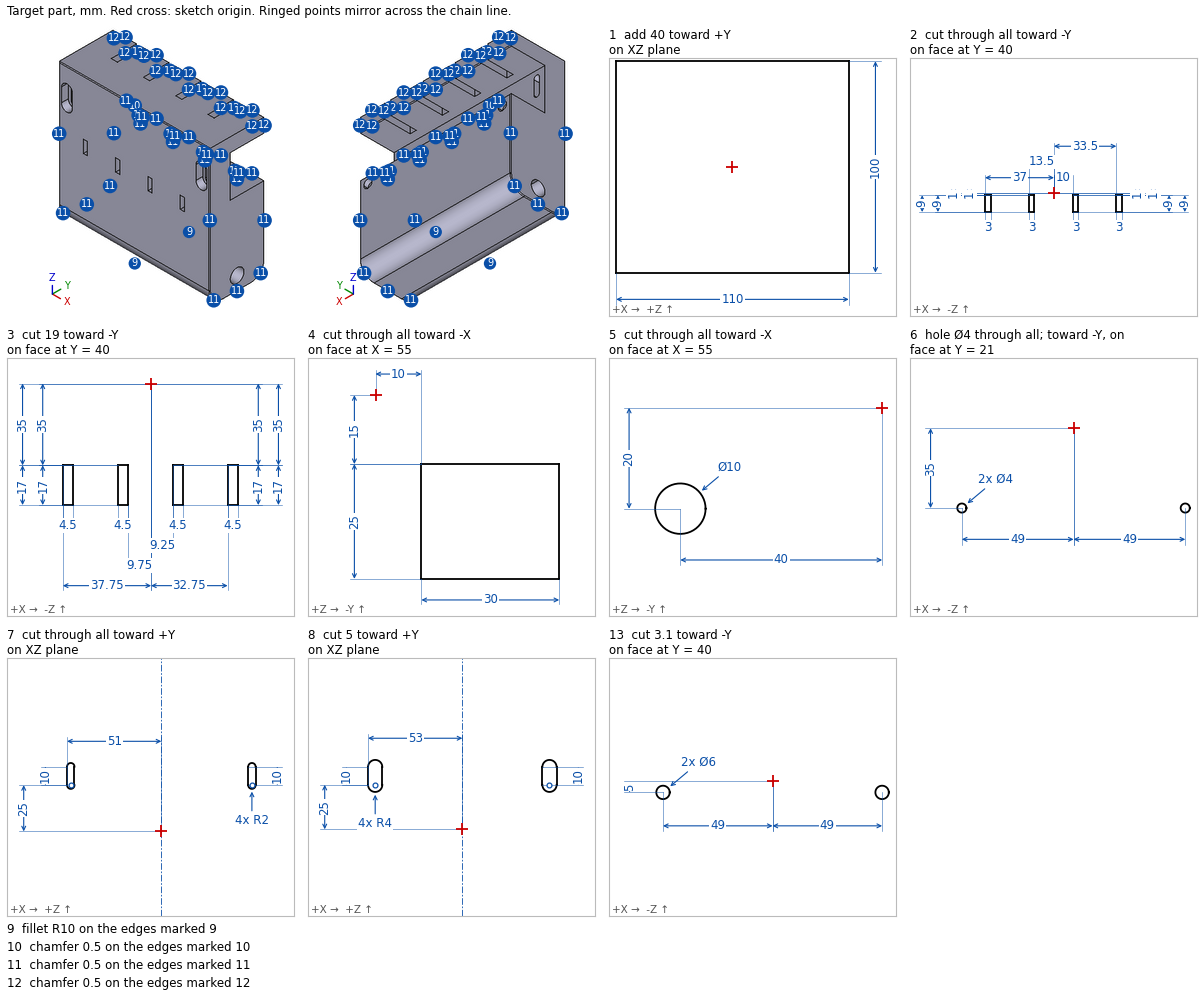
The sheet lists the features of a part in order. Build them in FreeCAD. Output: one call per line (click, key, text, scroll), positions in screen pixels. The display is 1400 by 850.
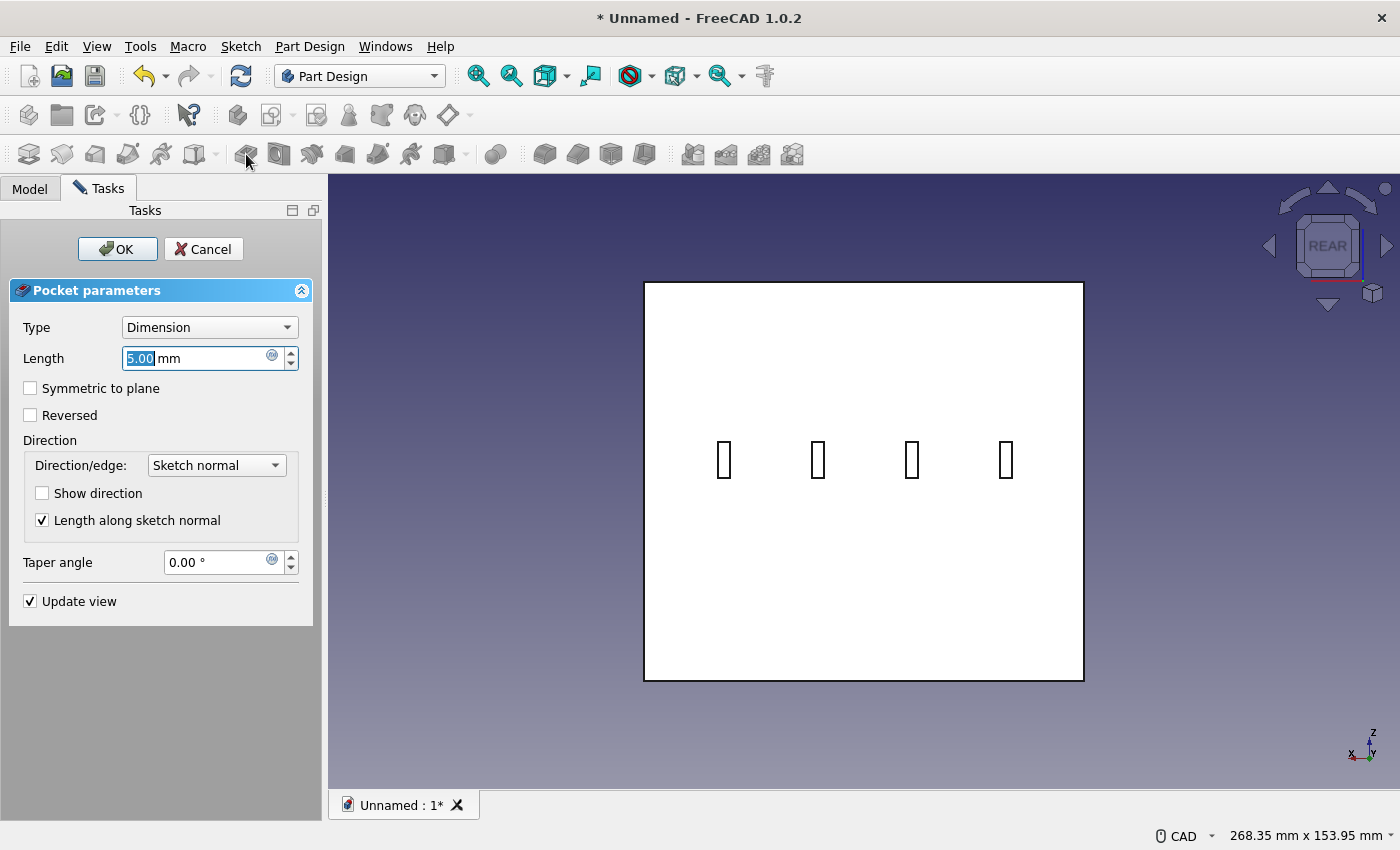
click(210, 328)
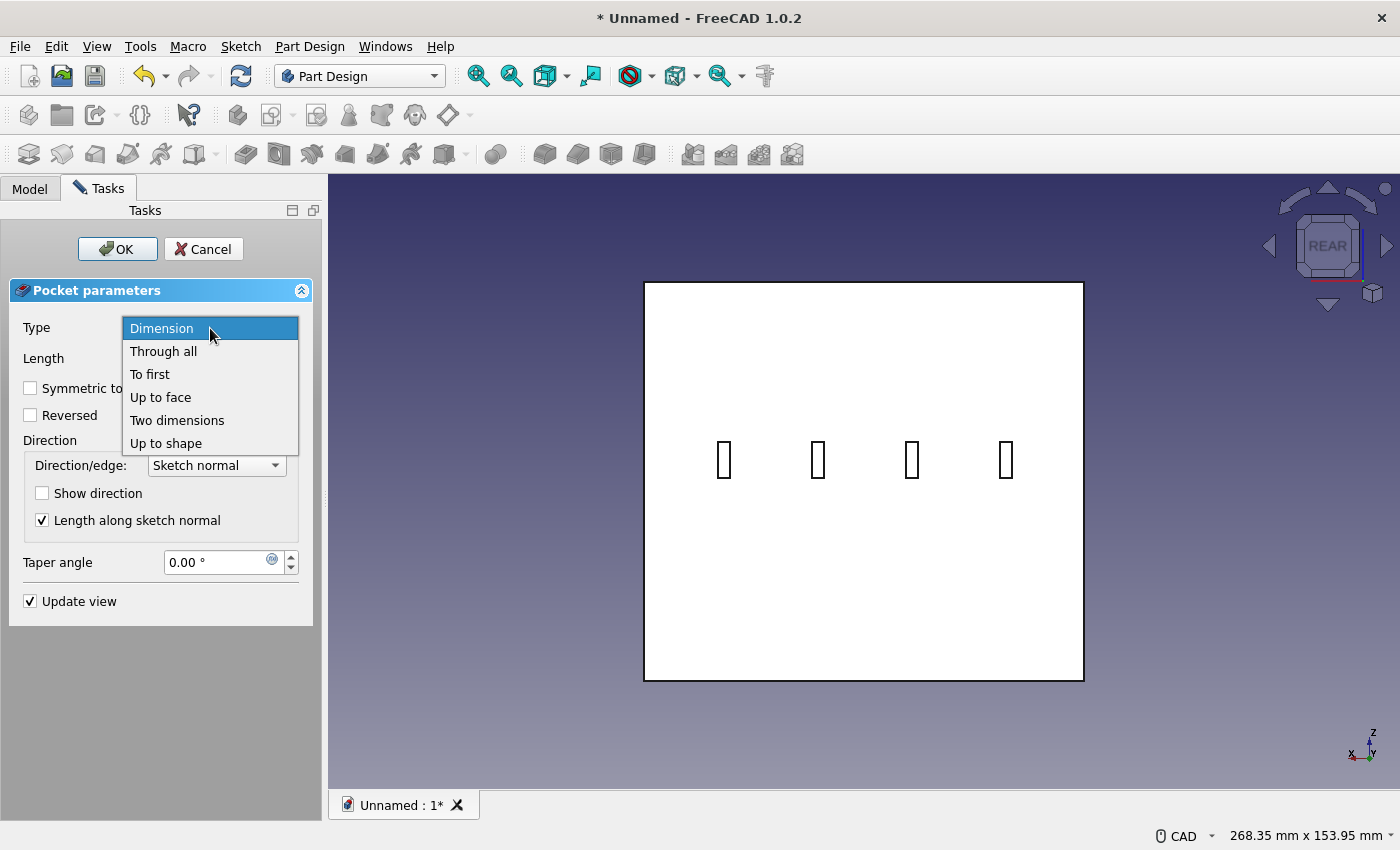
click(208, 352)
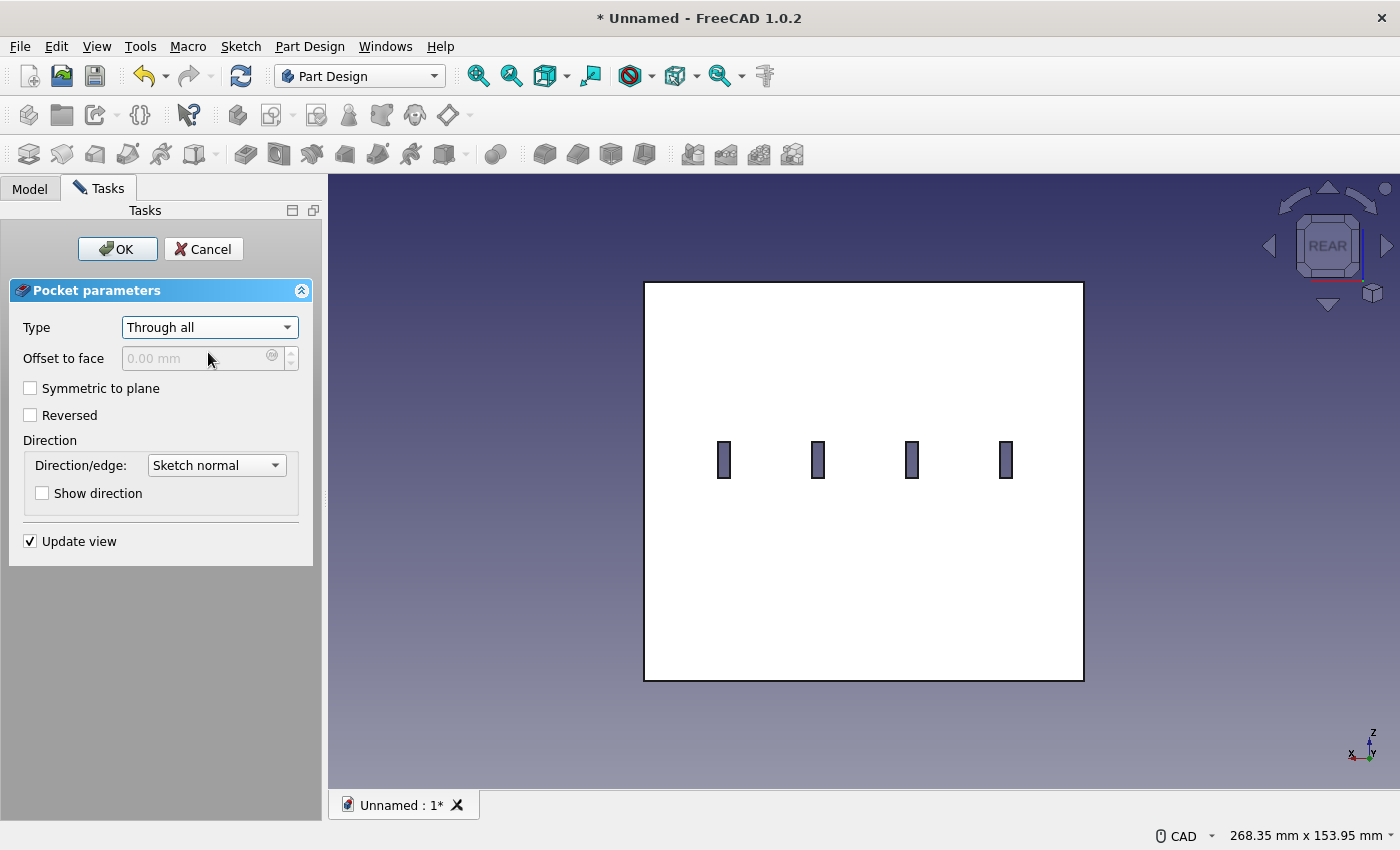
click(118, 249)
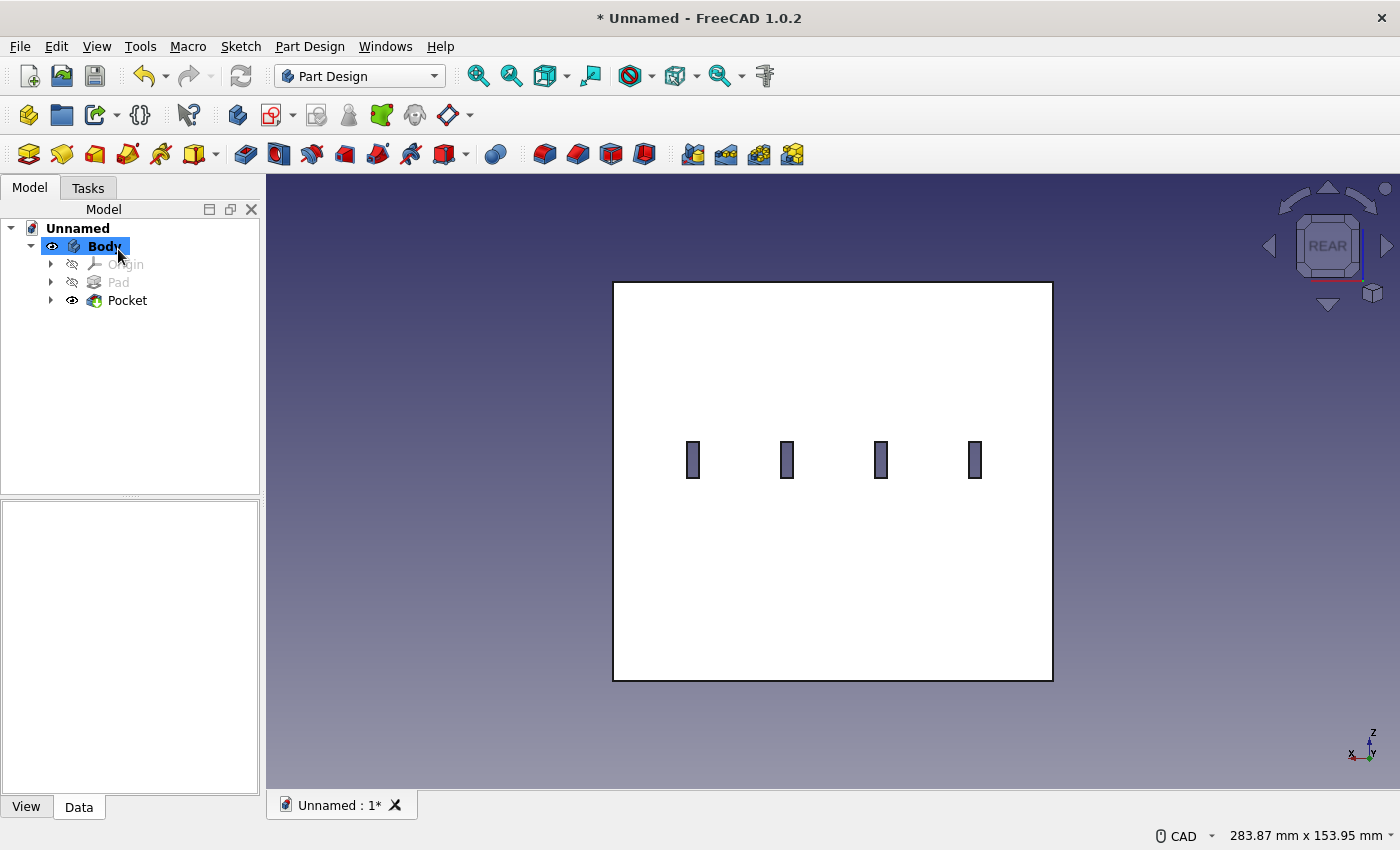
click(707, 595)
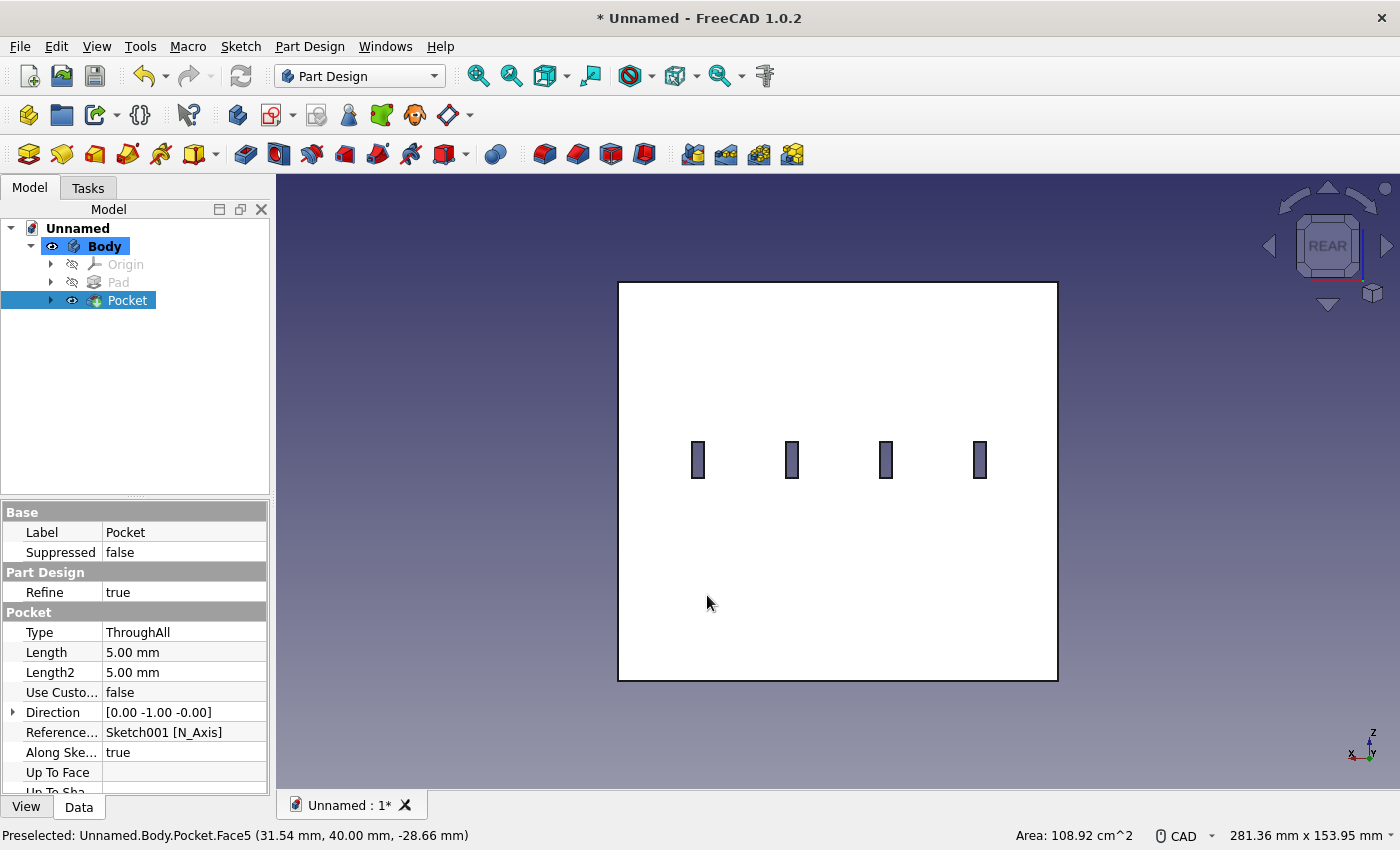
click(270, 116)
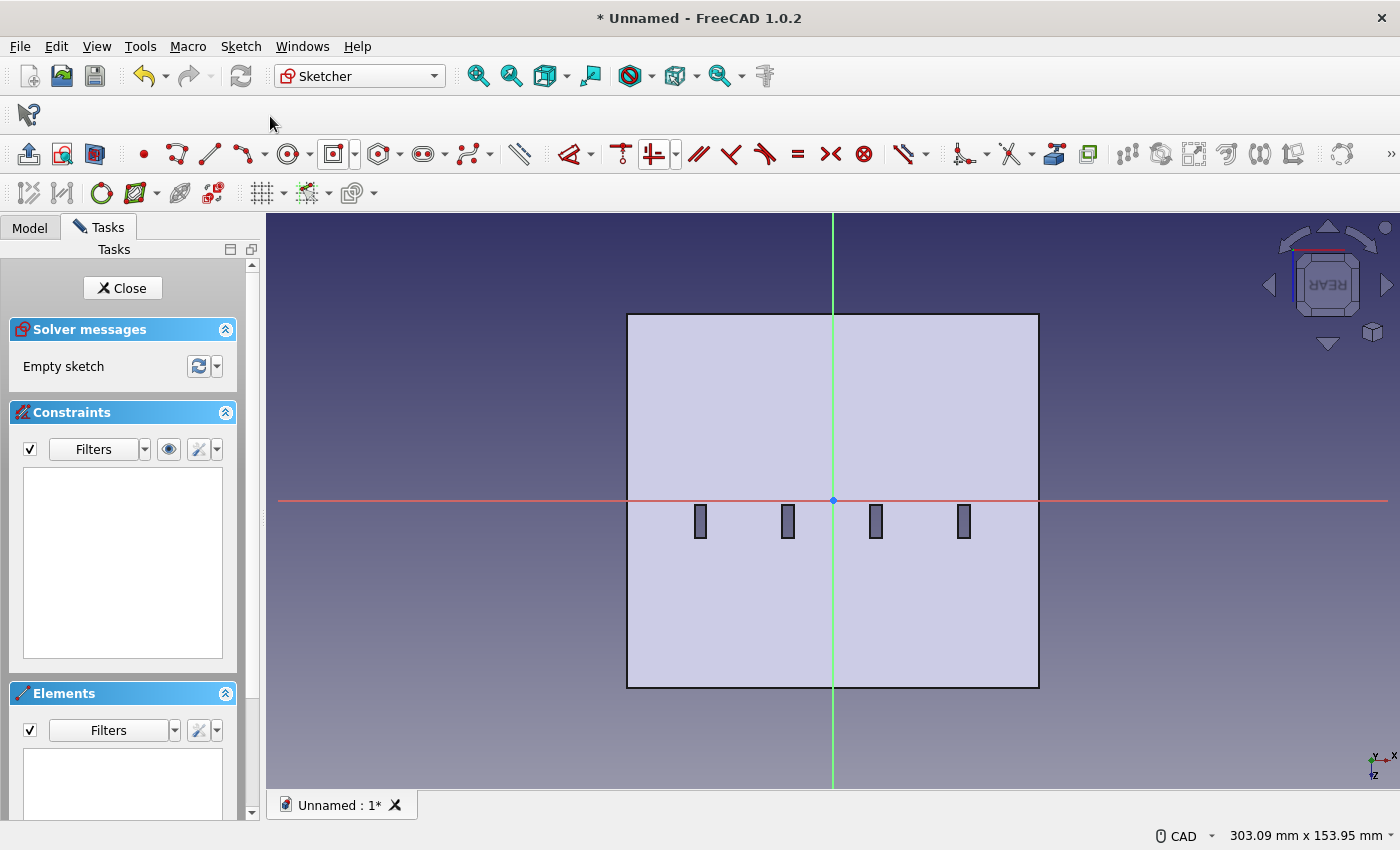
scroll(914, 717, up, 3)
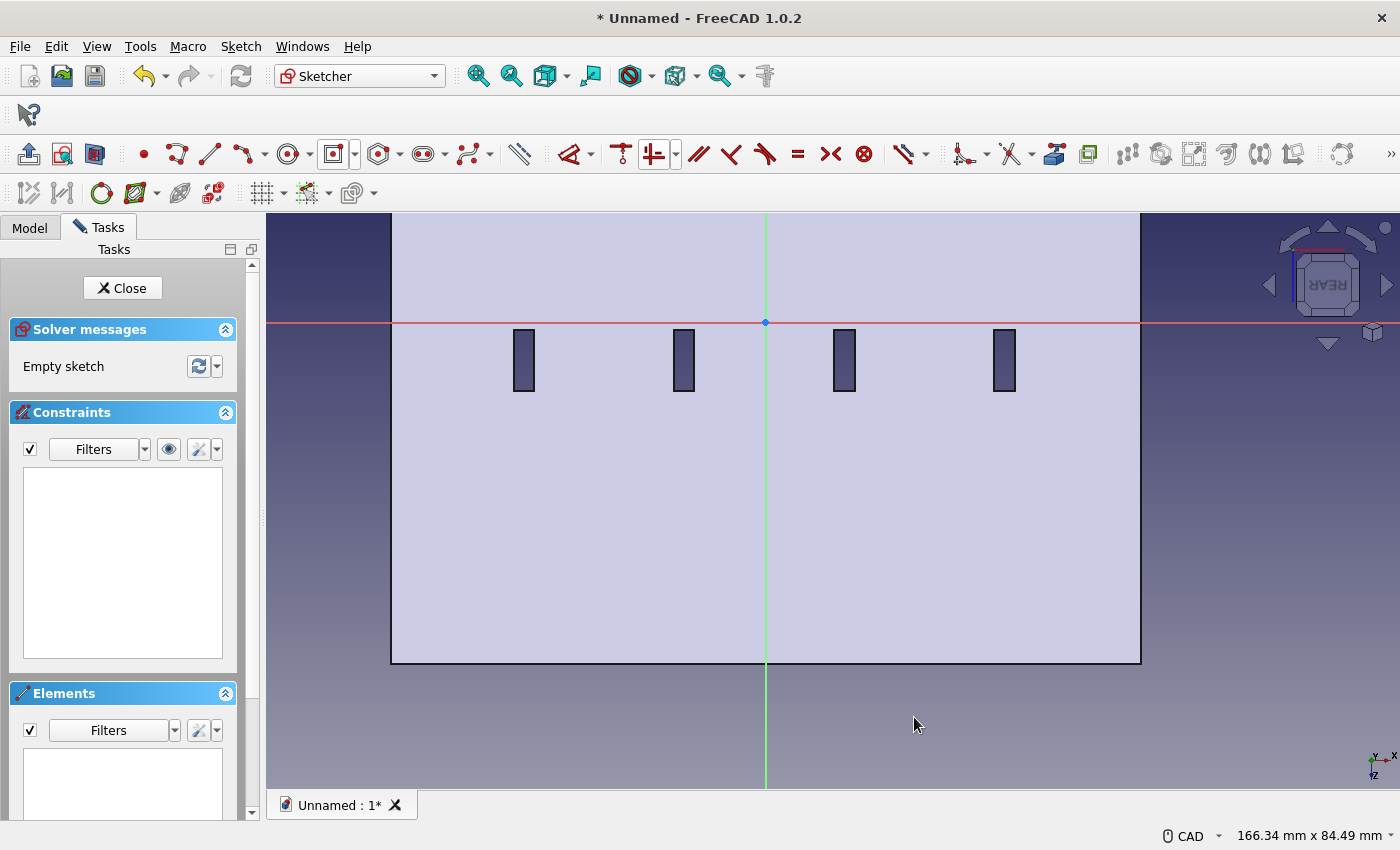
key(g)
key(r)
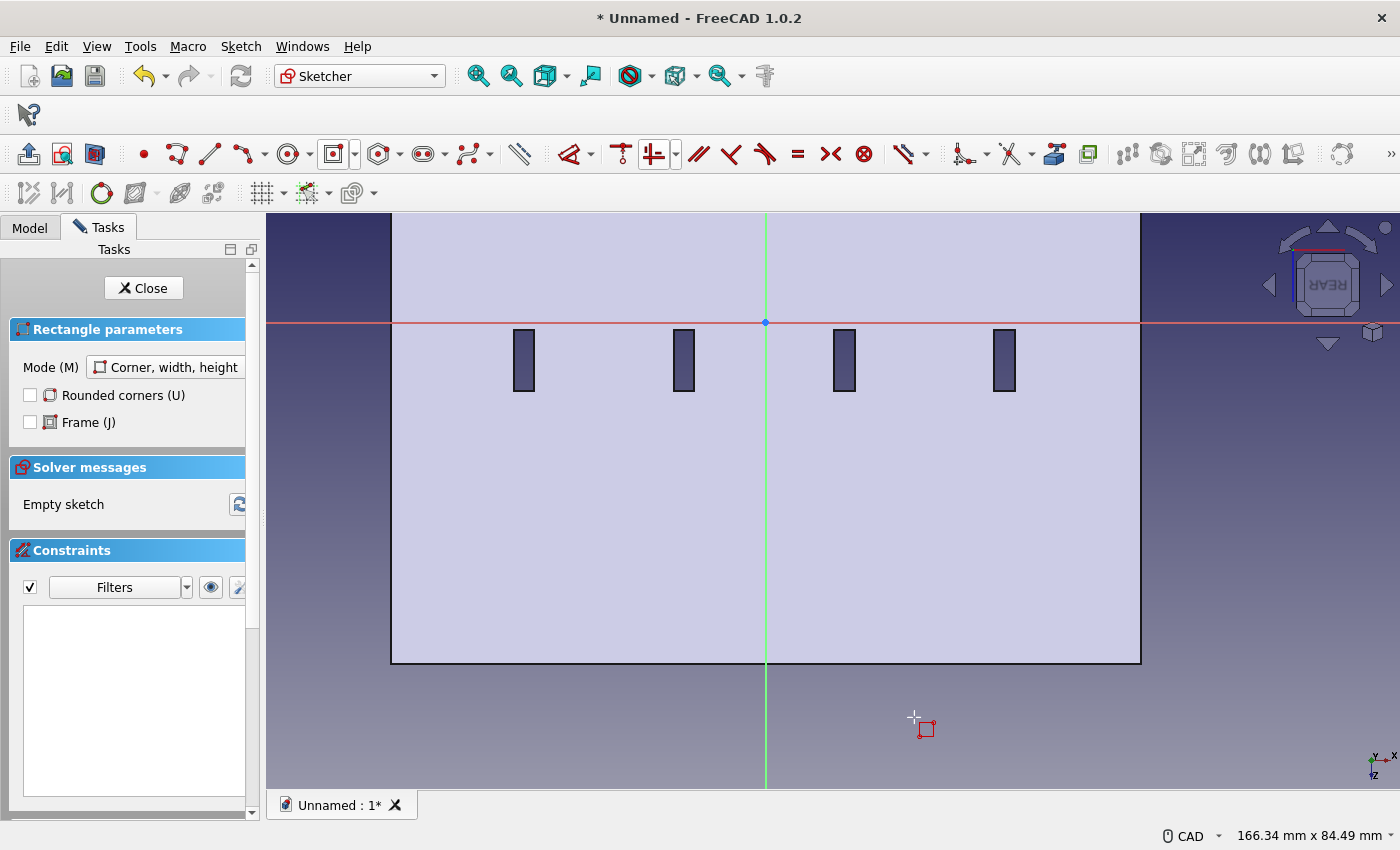
click(509, 561)
click(539, 677)